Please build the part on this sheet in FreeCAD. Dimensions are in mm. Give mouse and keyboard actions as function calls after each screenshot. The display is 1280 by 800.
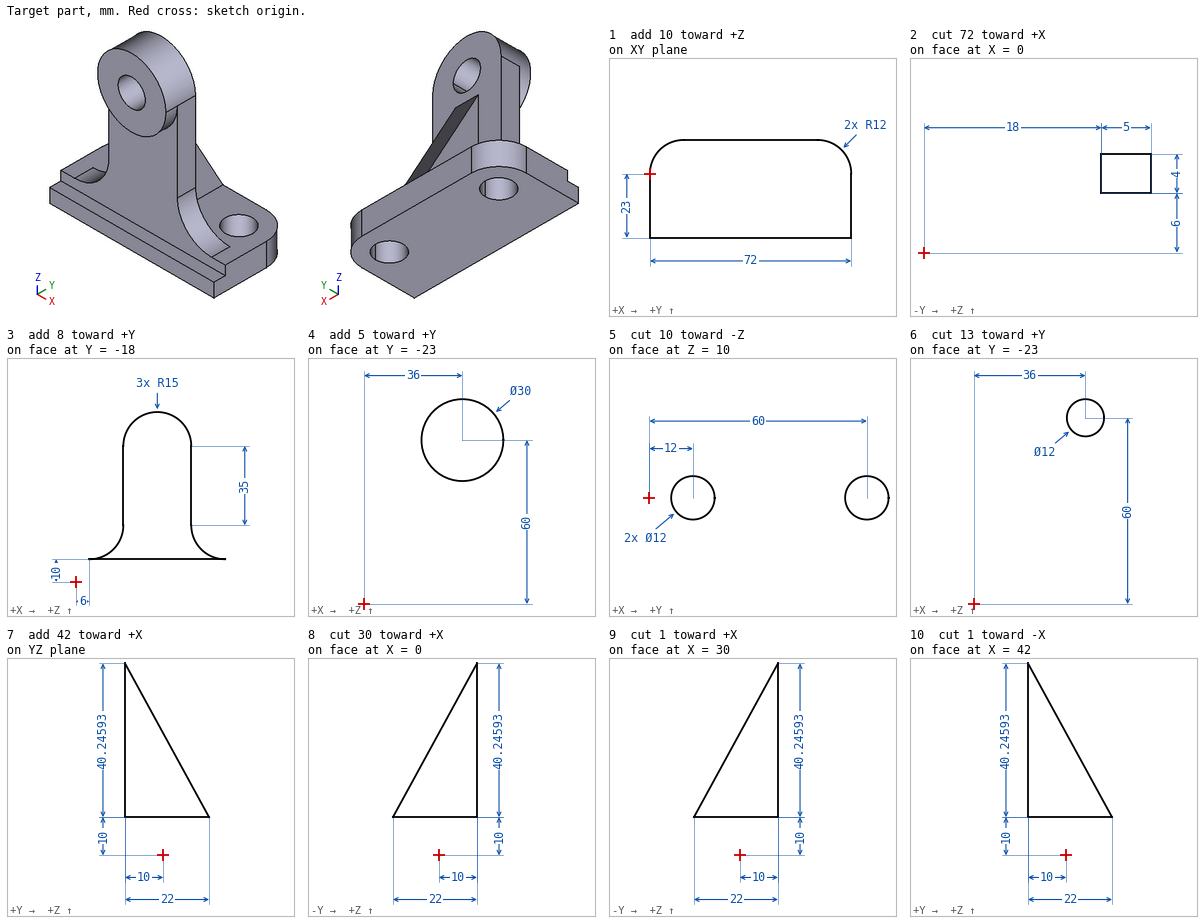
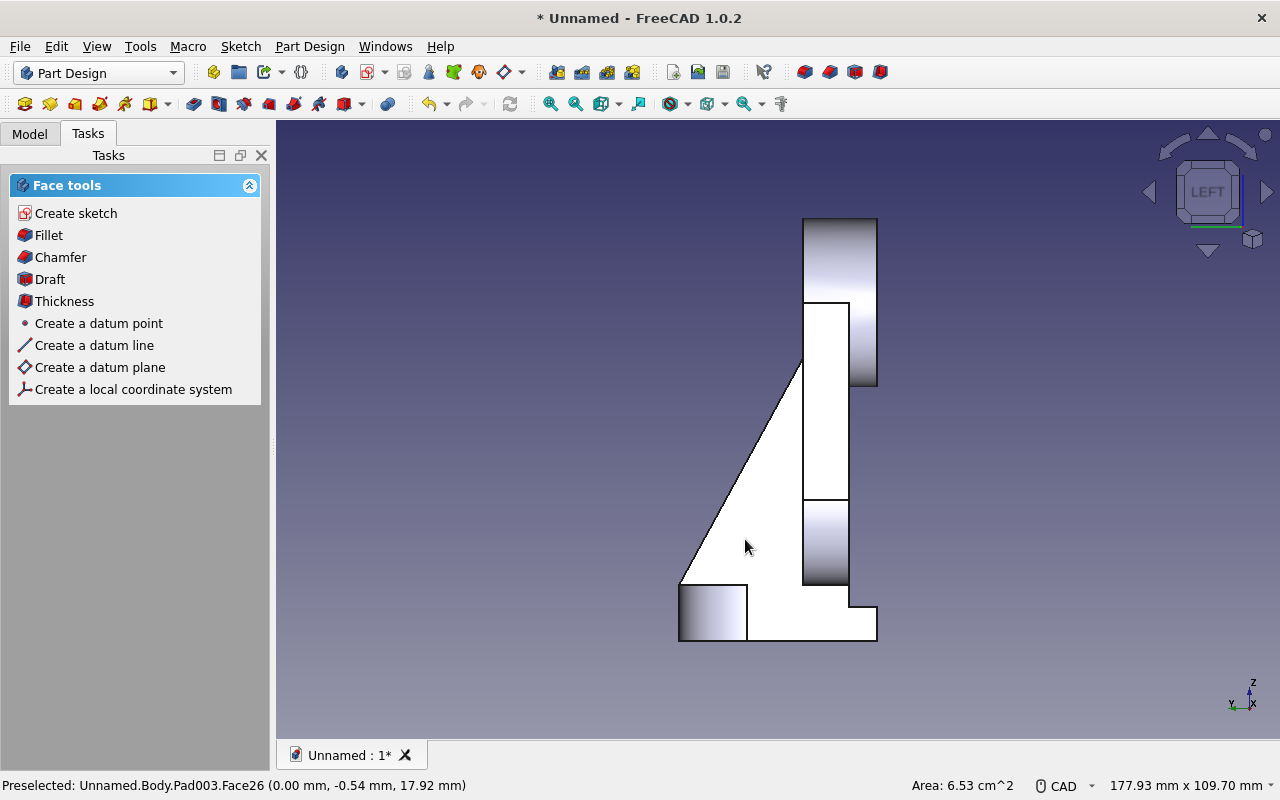
click(366, 72)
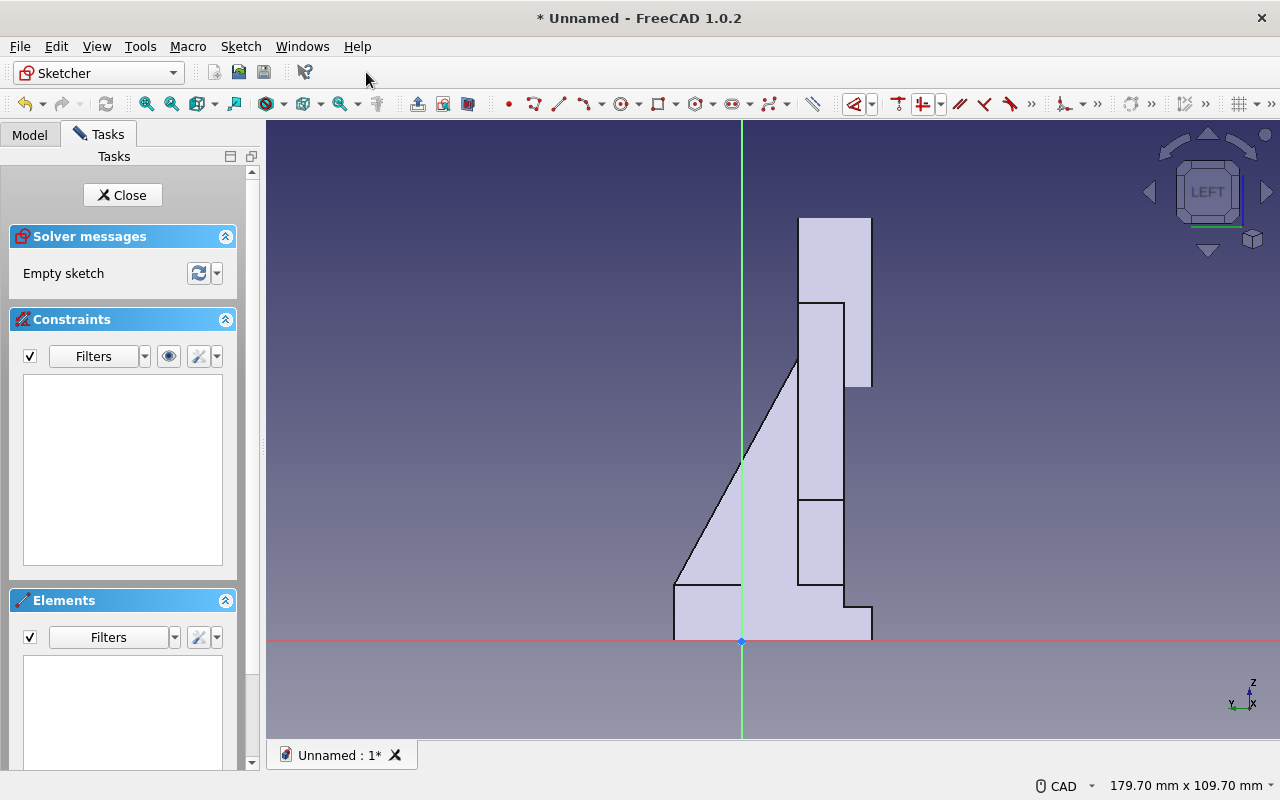
scroll(801, 641, up, 2)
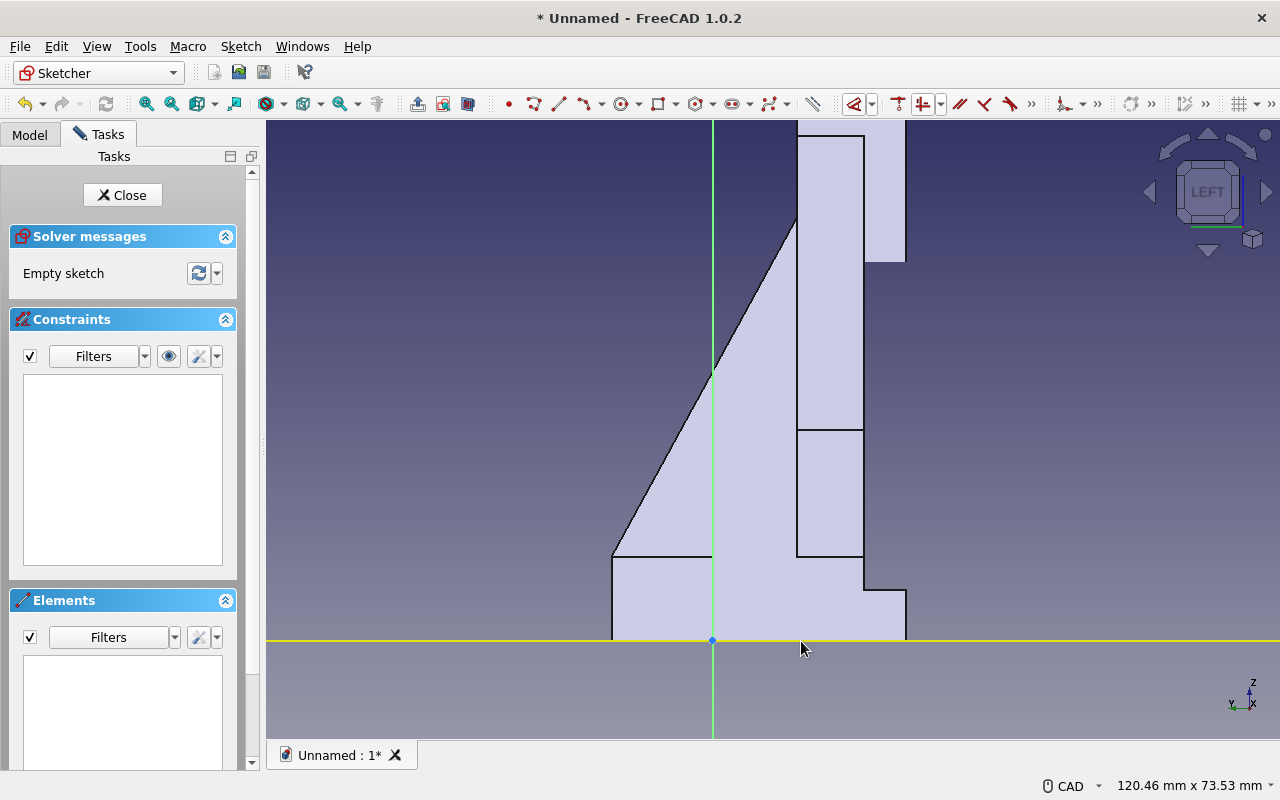
click(534, 104)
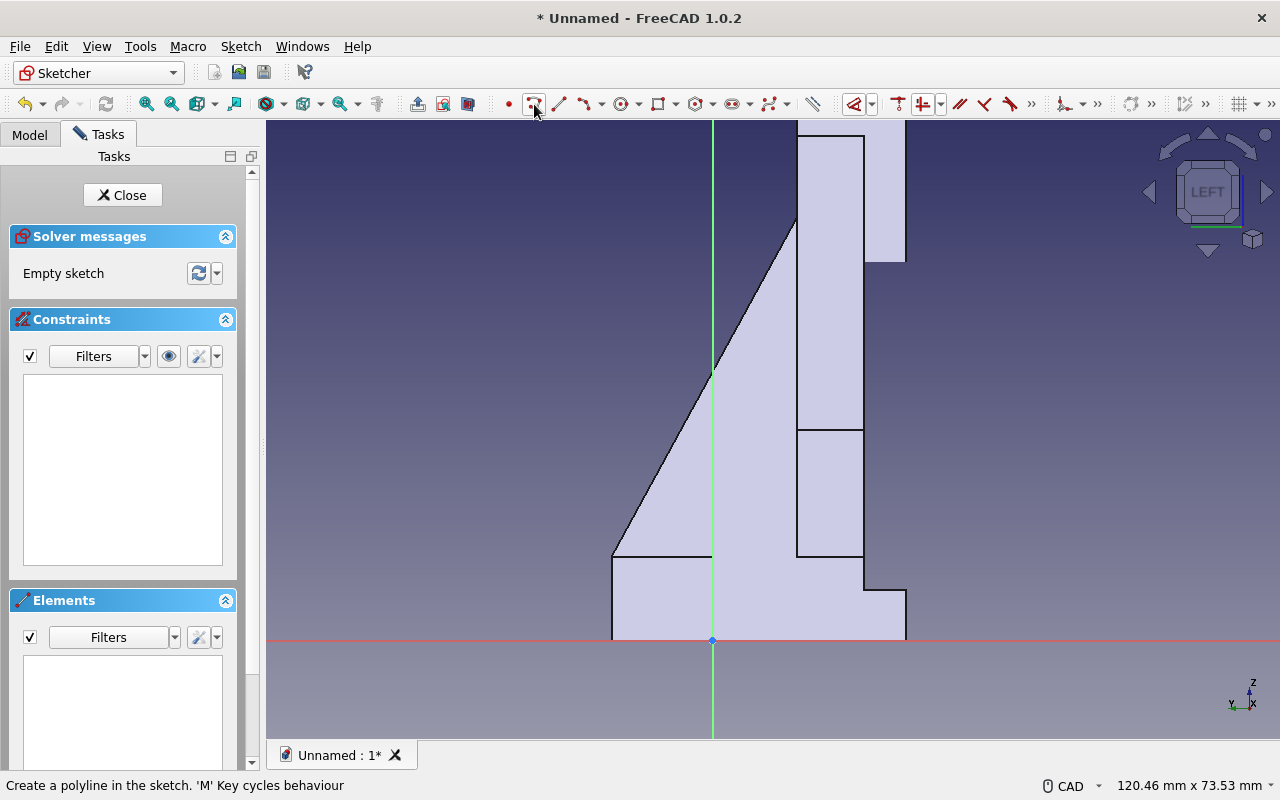
click(797, 557)
click(797, 218)
click(612, 557)
click(797, 558)
key(Escape)
key(Escape)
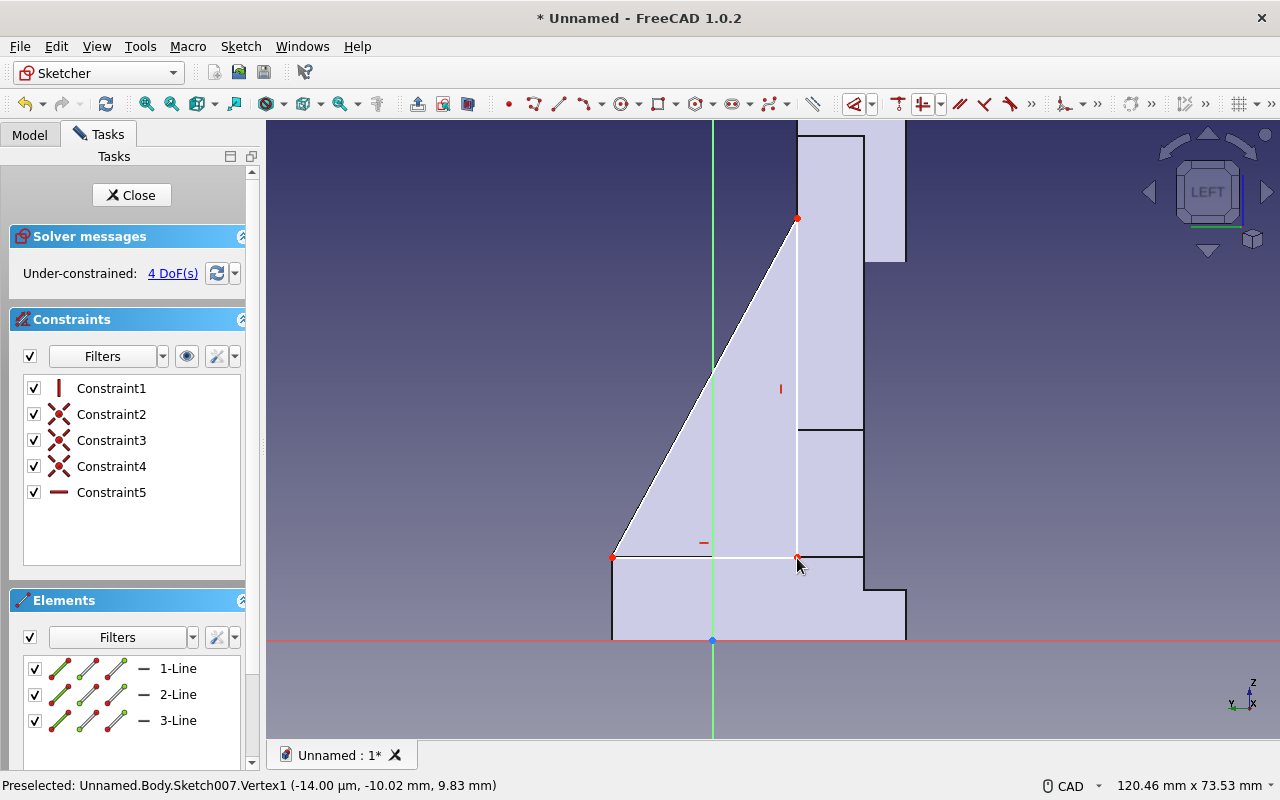
click(667, 558)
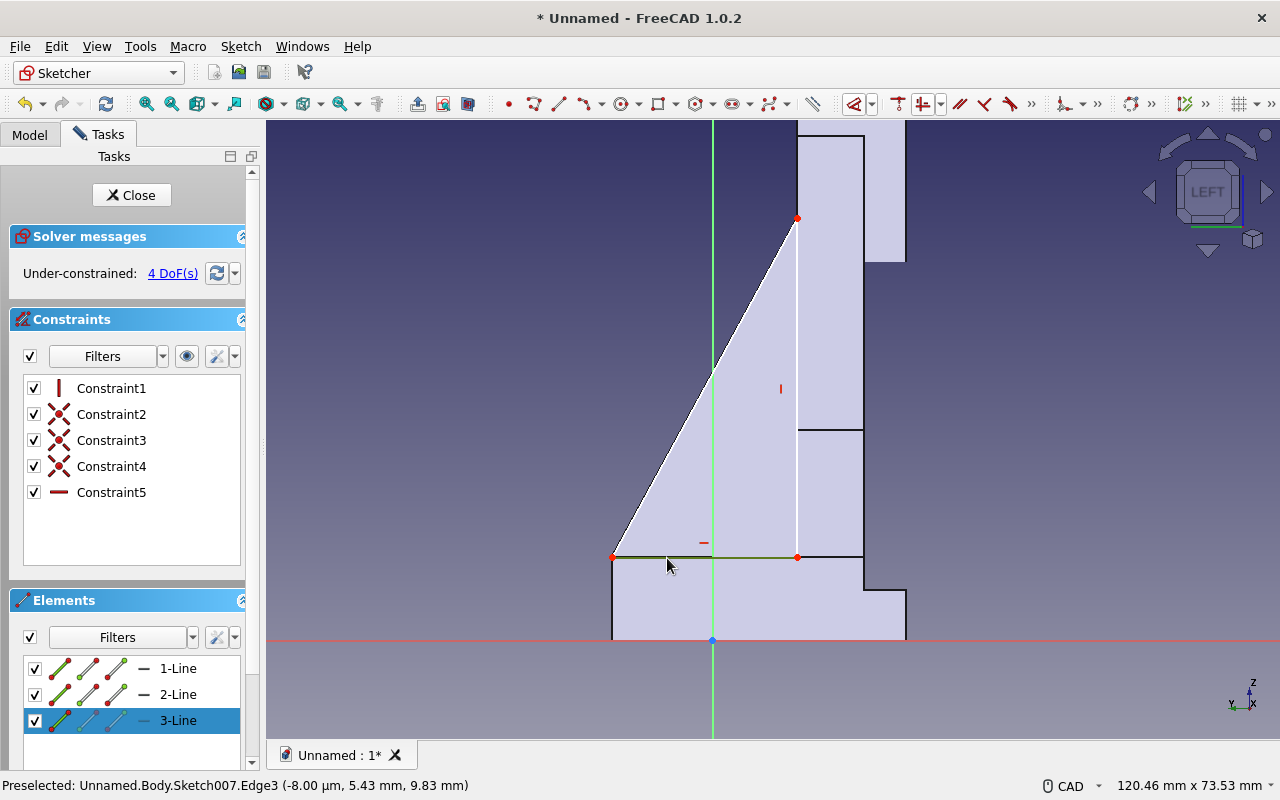
click(872, 104)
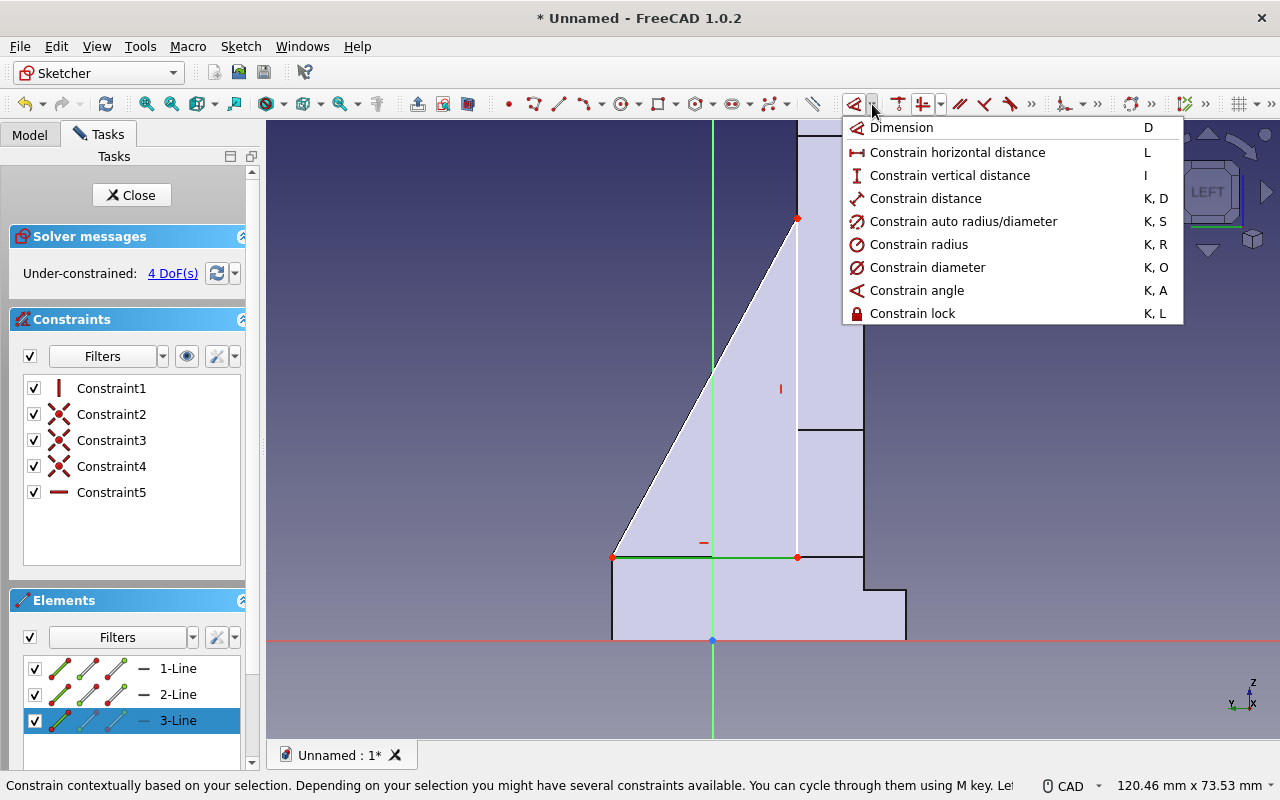
click(1013, 152)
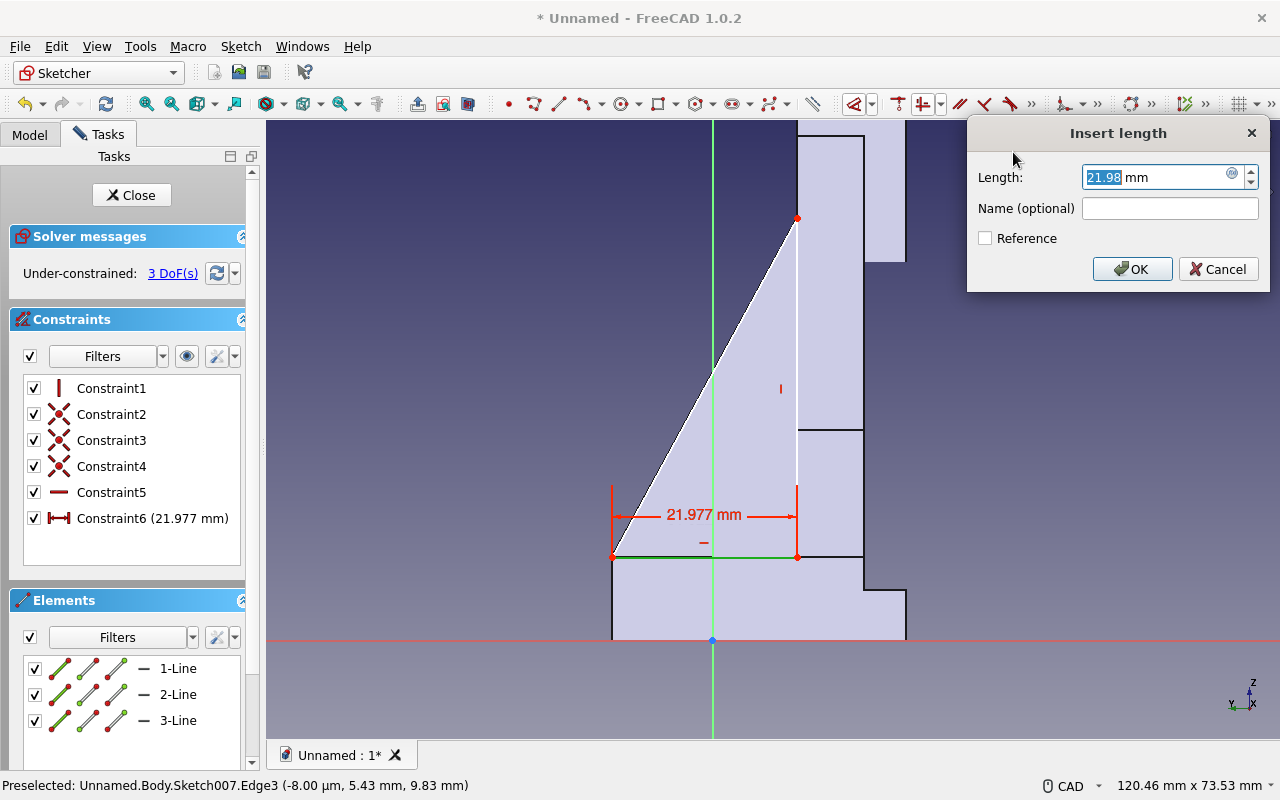
text(22)
key(Return)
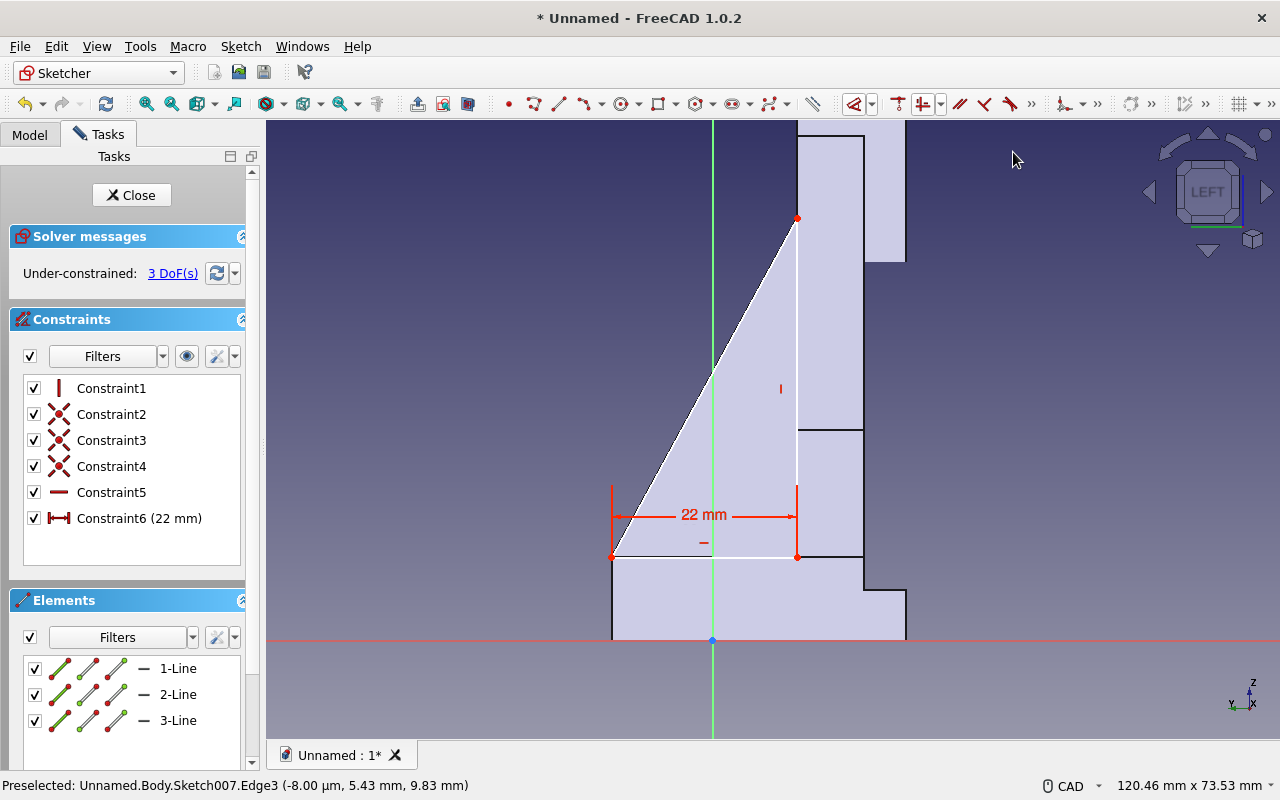
click(797, 558)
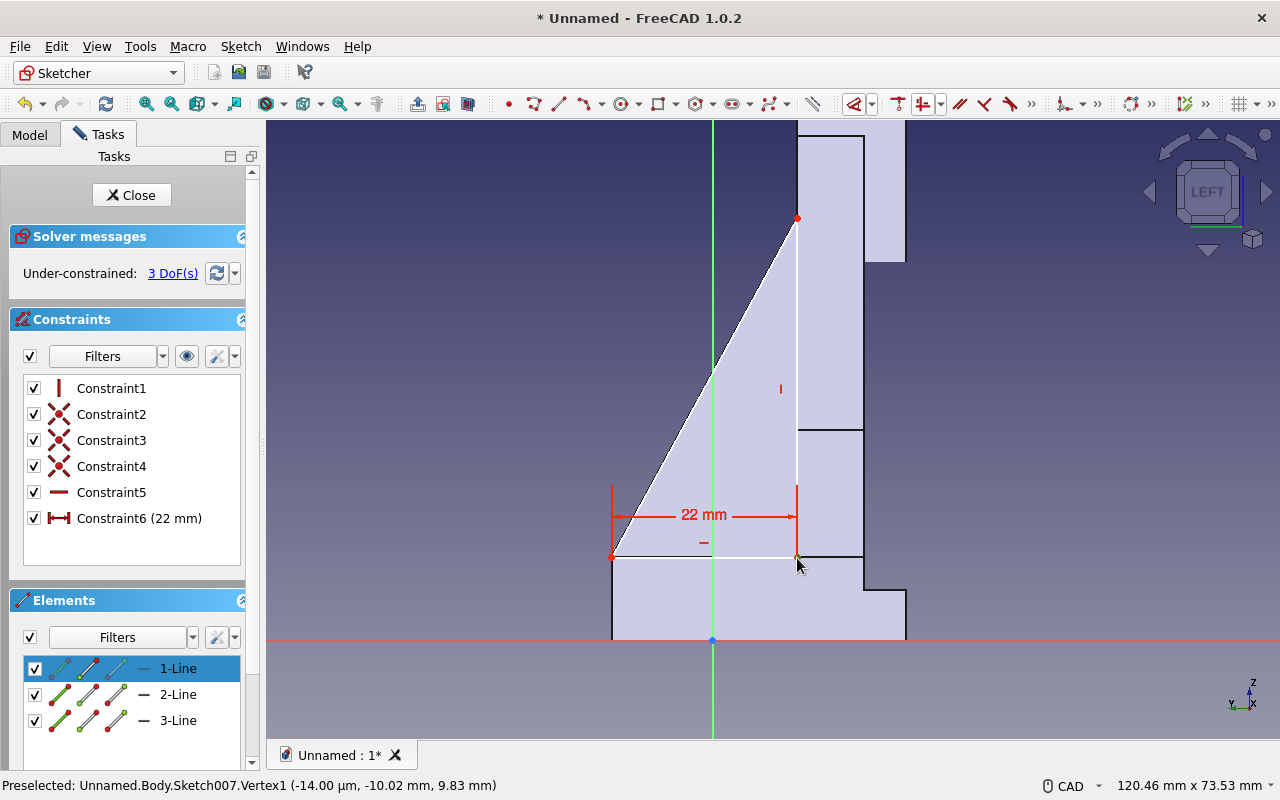
click(872, 104)